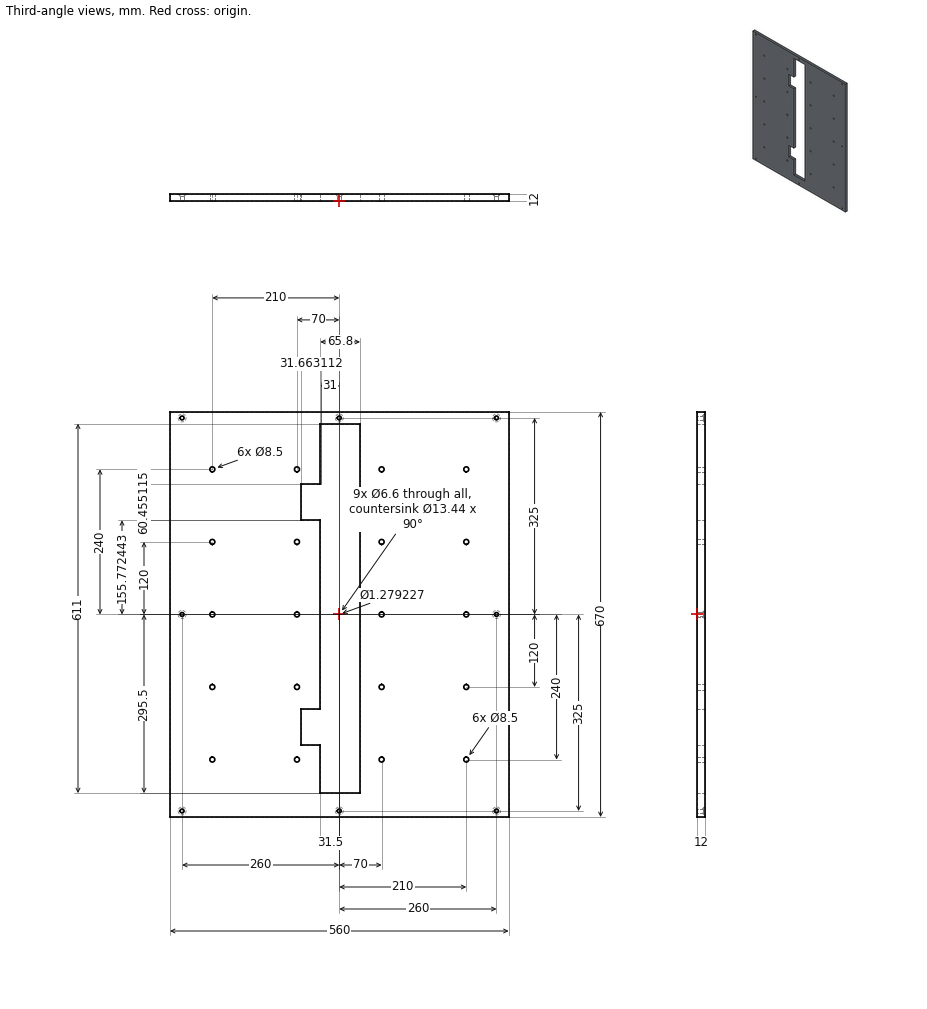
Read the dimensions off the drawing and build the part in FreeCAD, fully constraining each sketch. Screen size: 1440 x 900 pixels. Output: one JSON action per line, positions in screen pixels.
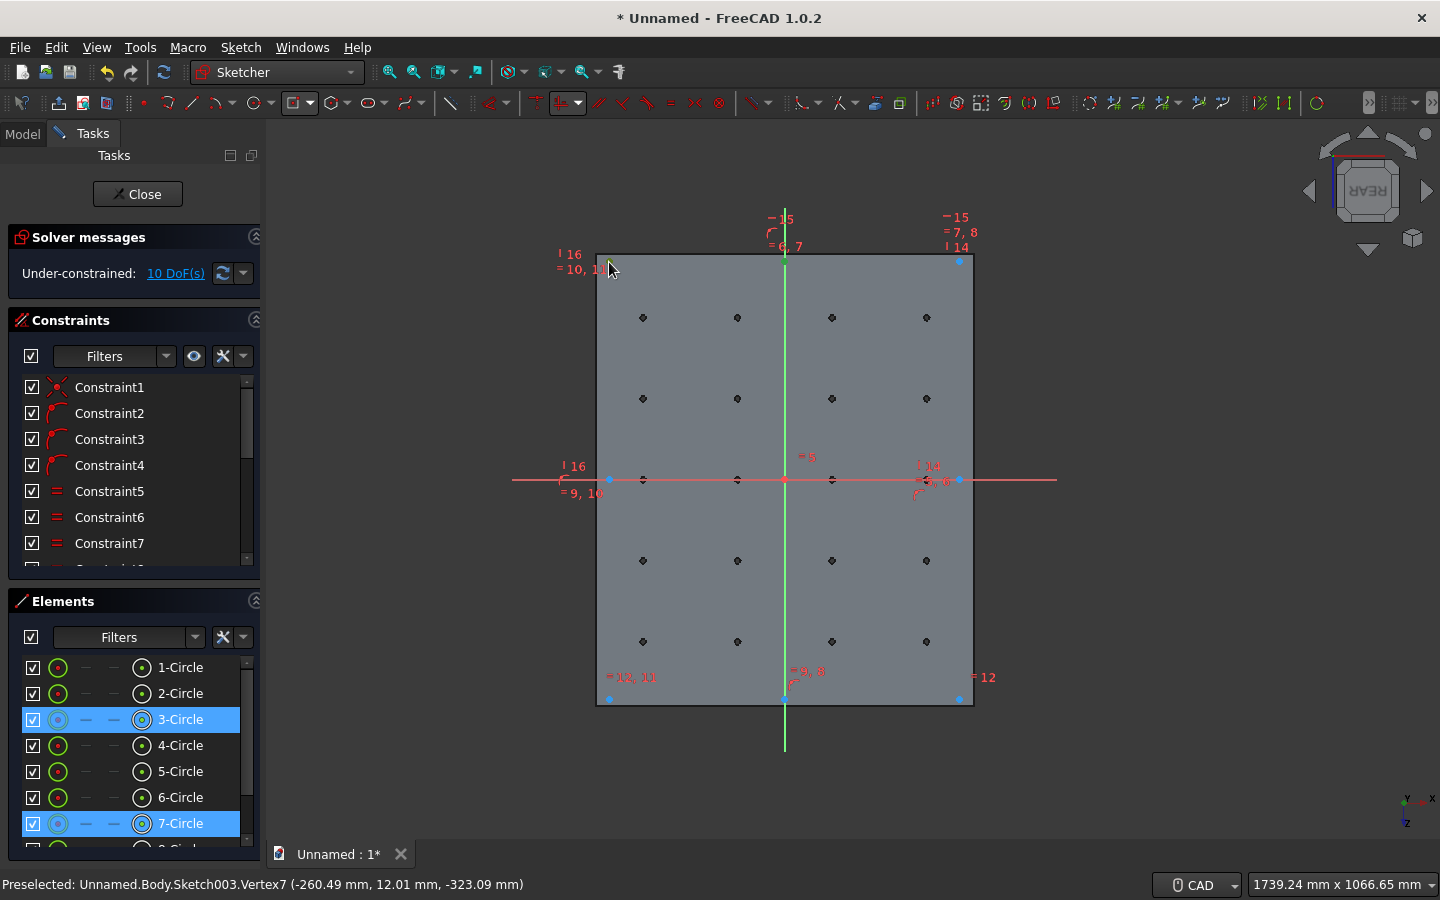
{"action": "left_click", "coordinate": [580, 104]}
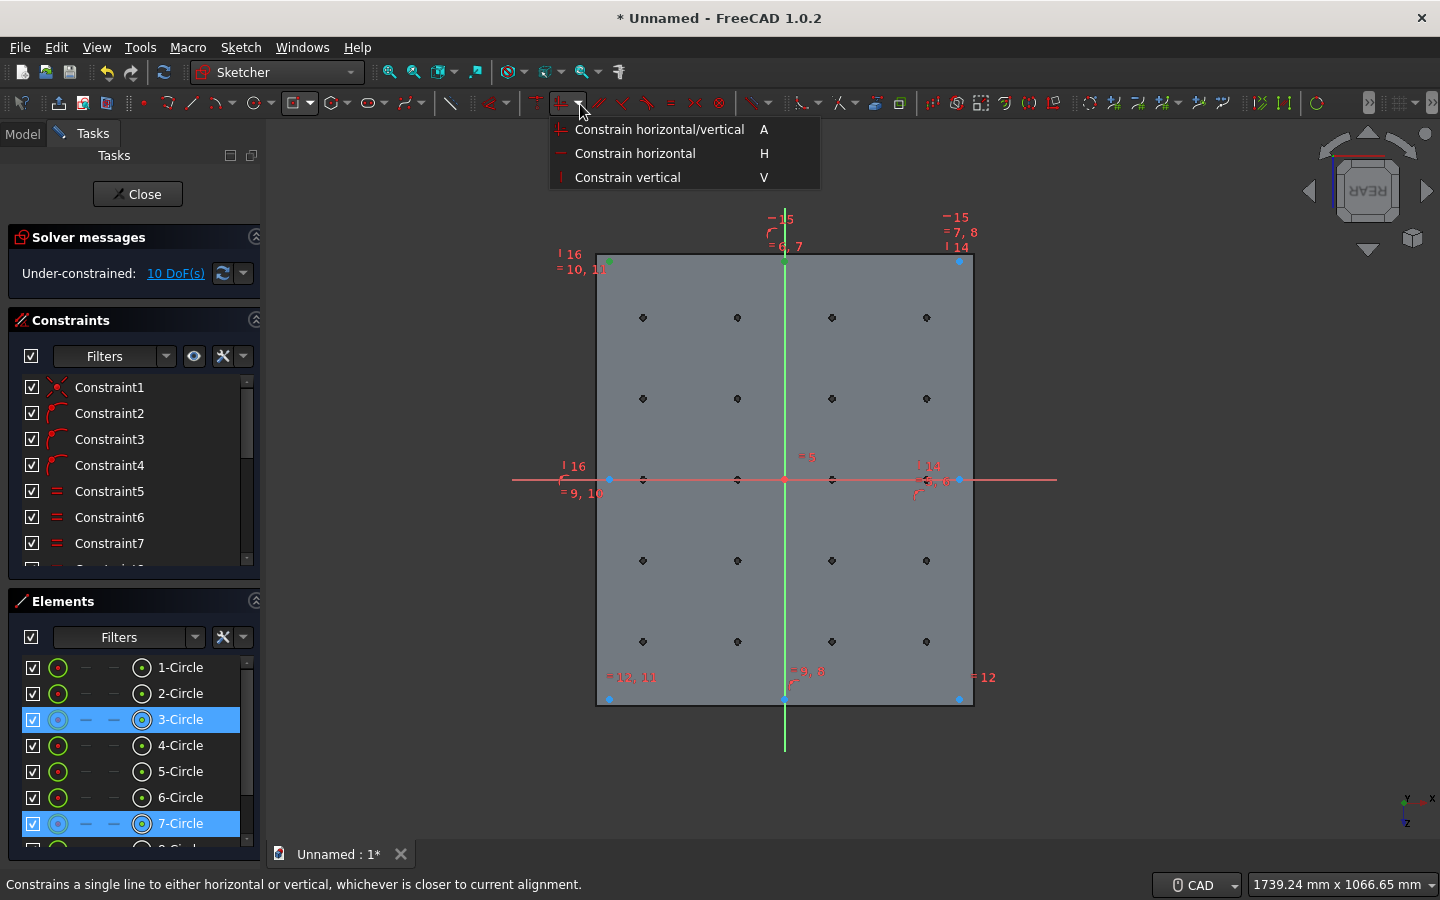
{"action": "left_click", "coordinate": [685, 153]}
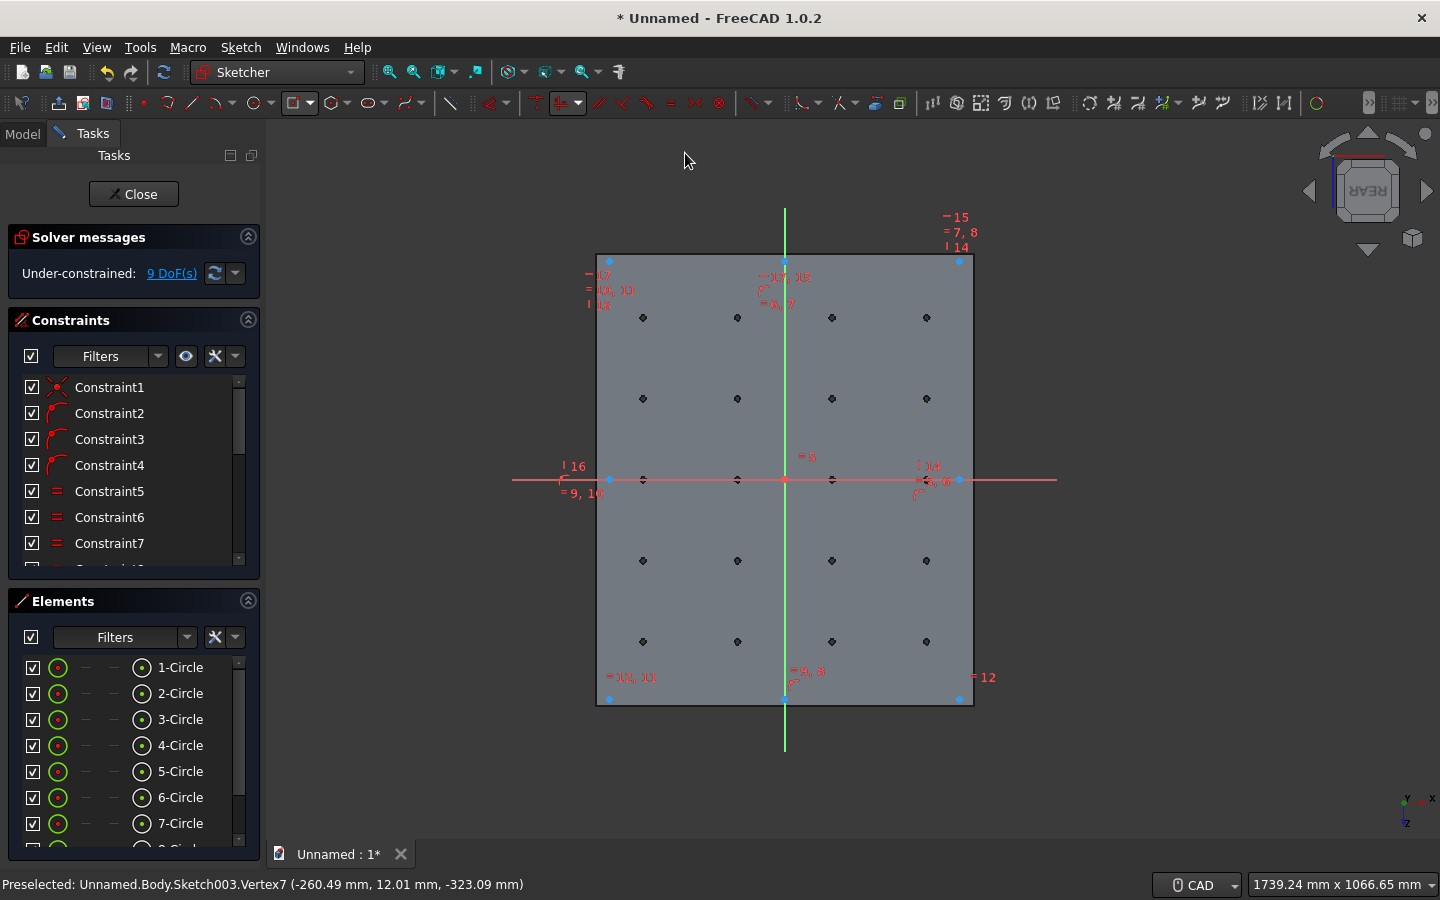
{"action": "left_click", "coordinate": [609, 480]}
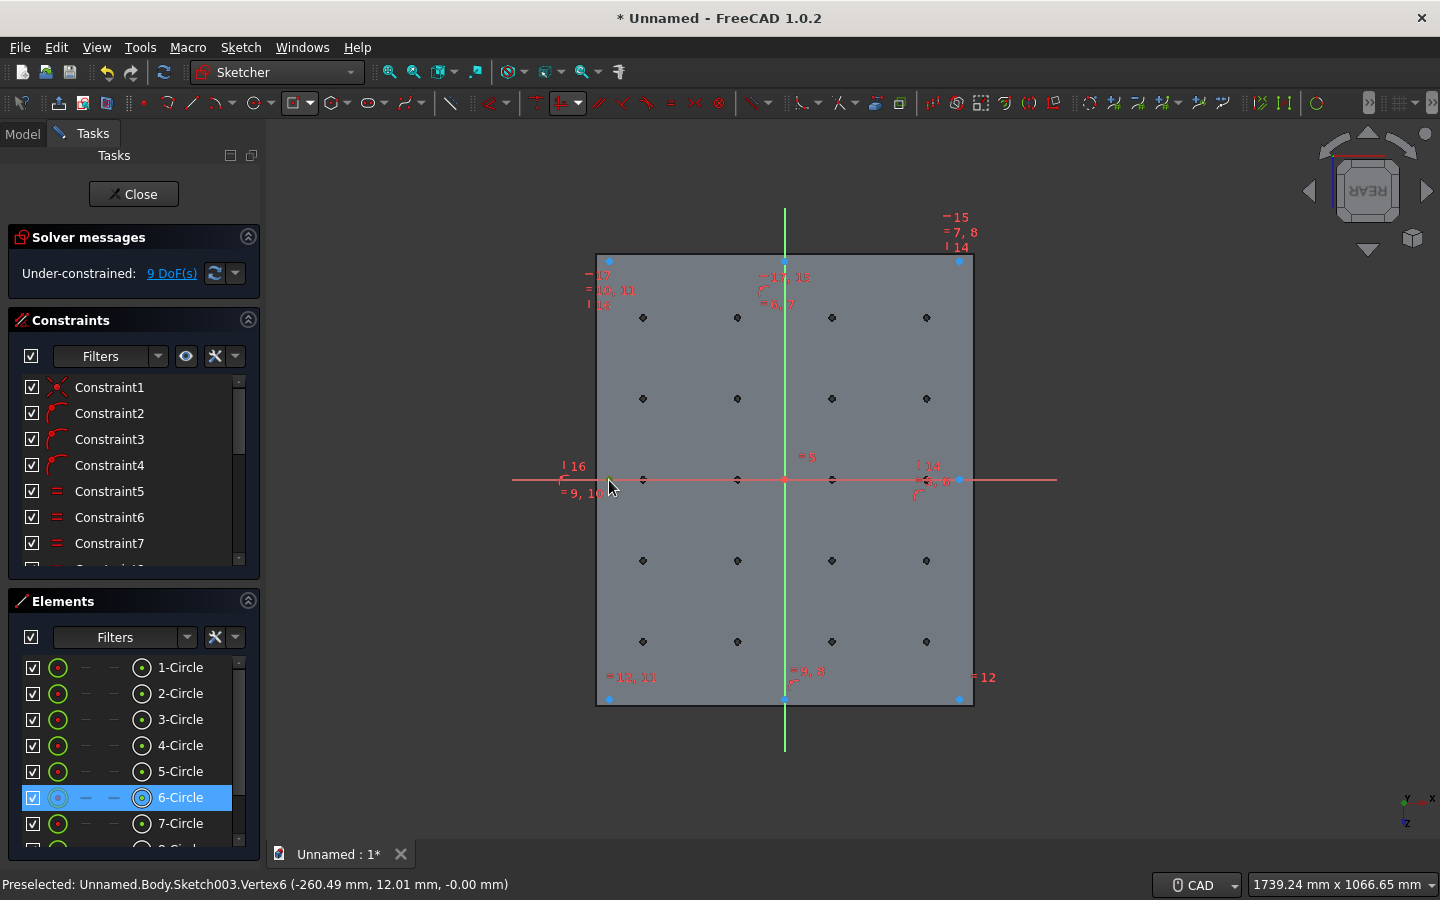
{"action": "left_click", "coordinate": [609, 700]}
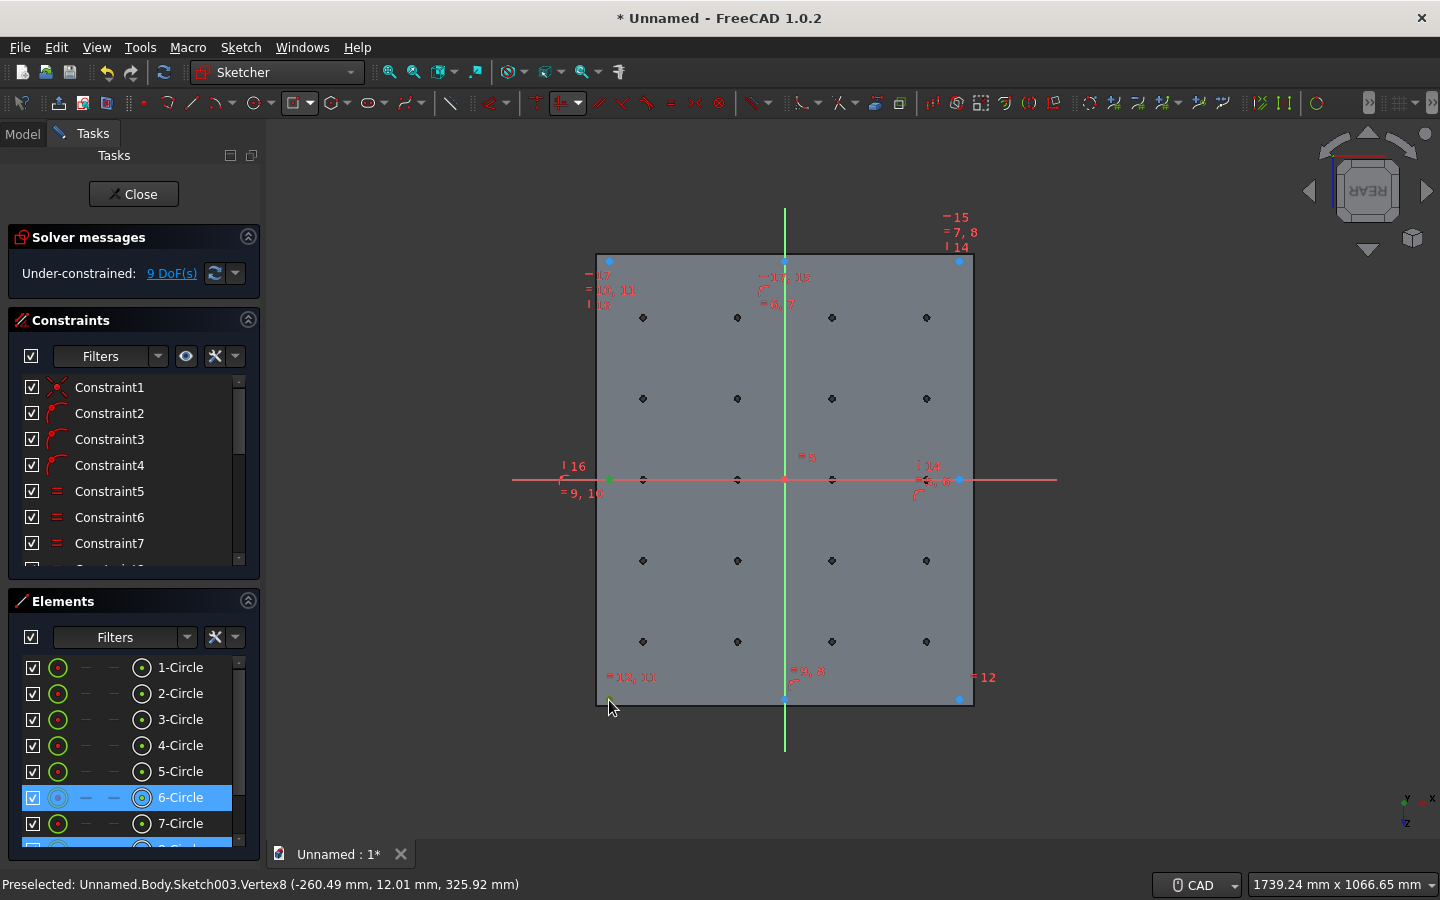
{"action": "left_click", "coordinate": [580, 104]}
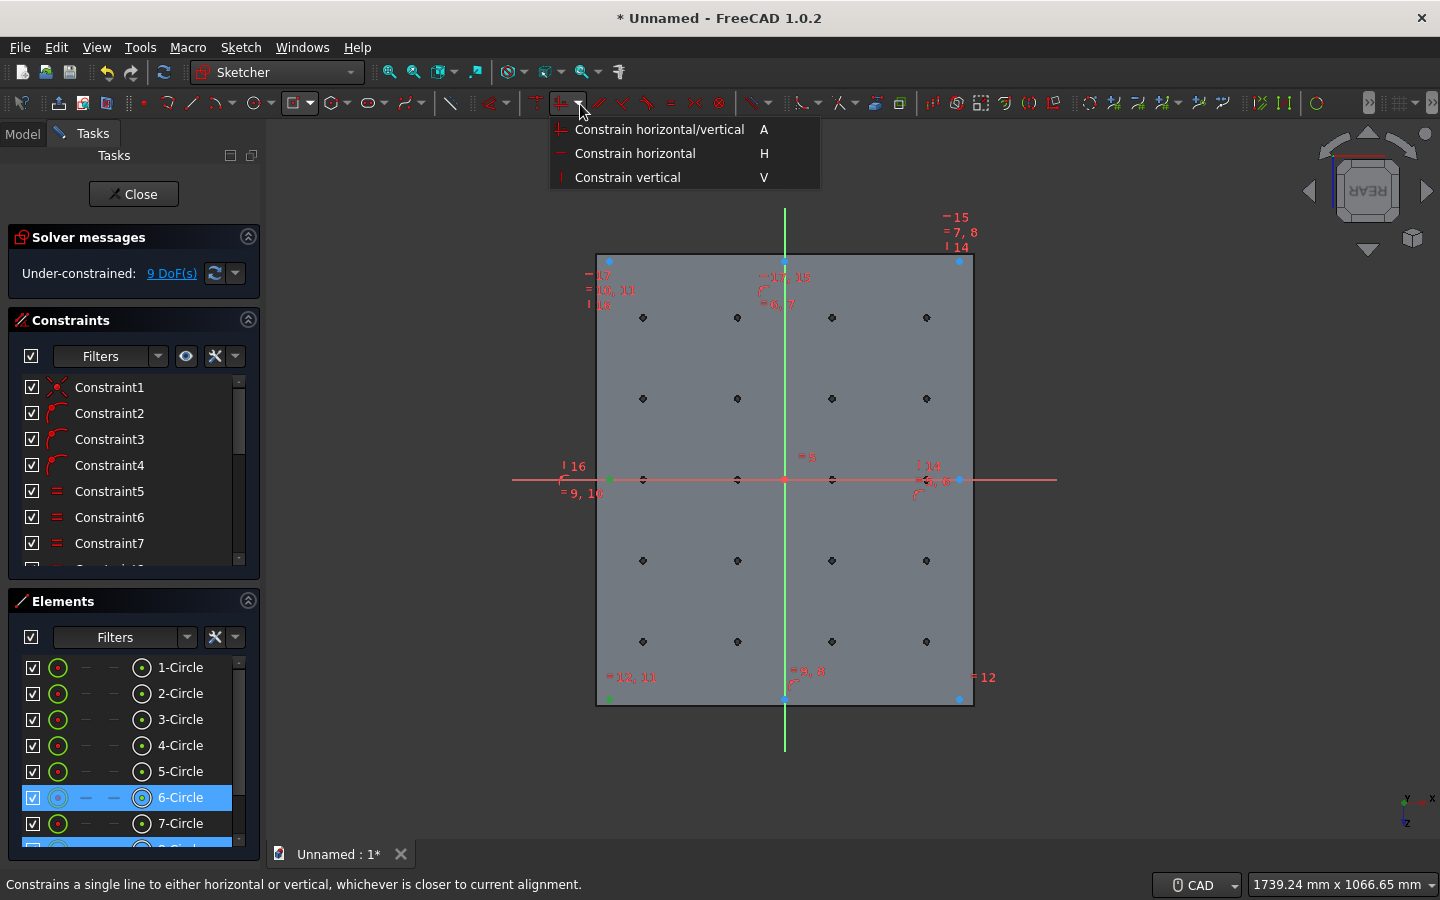
{"action": "left_click", "coordinate": [685, 177]}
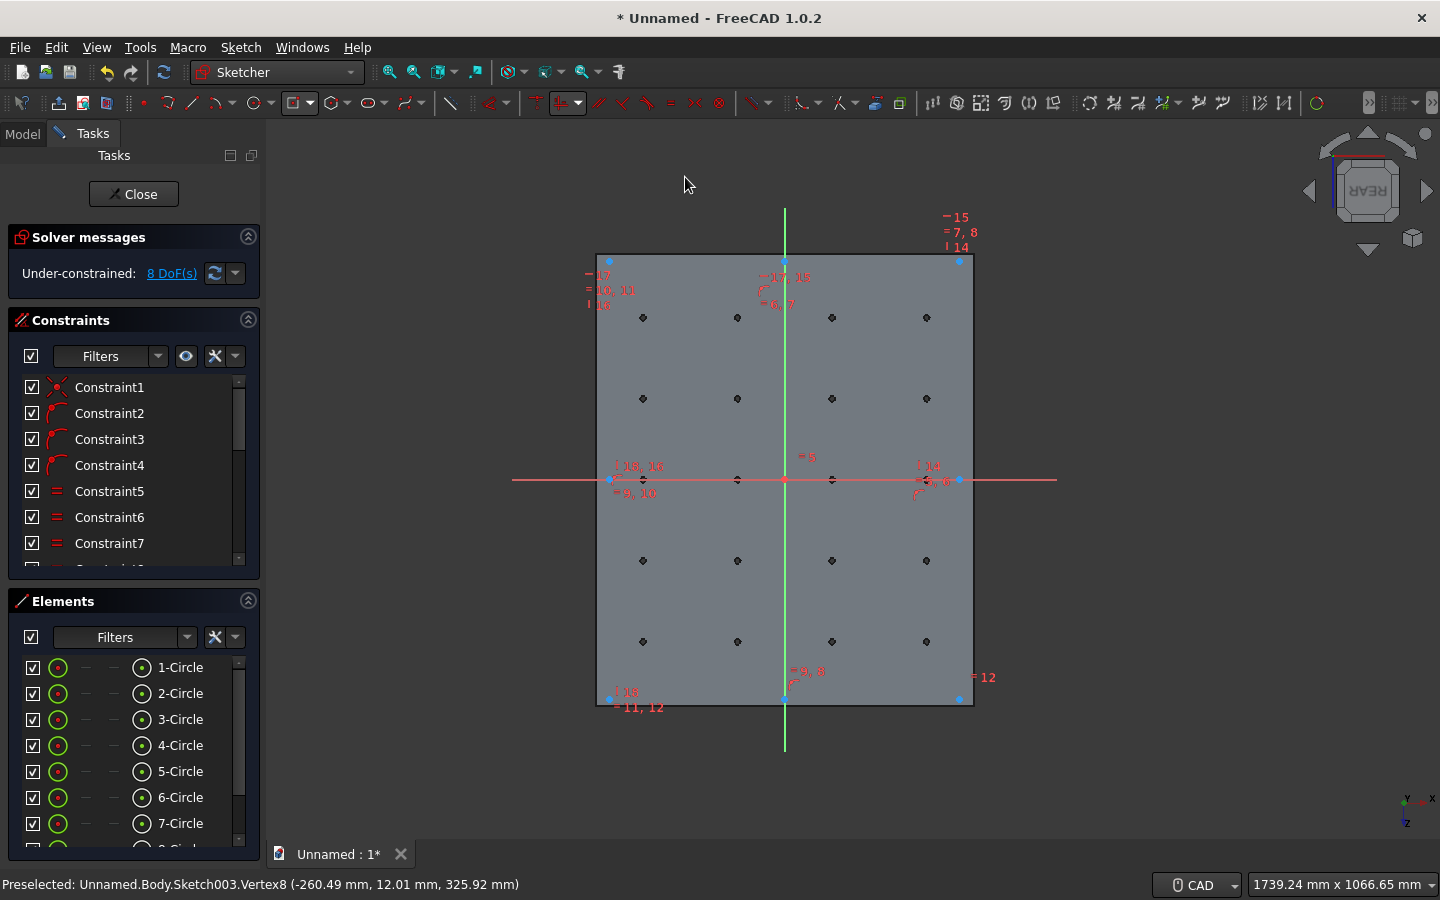
{"action": "left_click", "coordinate": [785, 700]}